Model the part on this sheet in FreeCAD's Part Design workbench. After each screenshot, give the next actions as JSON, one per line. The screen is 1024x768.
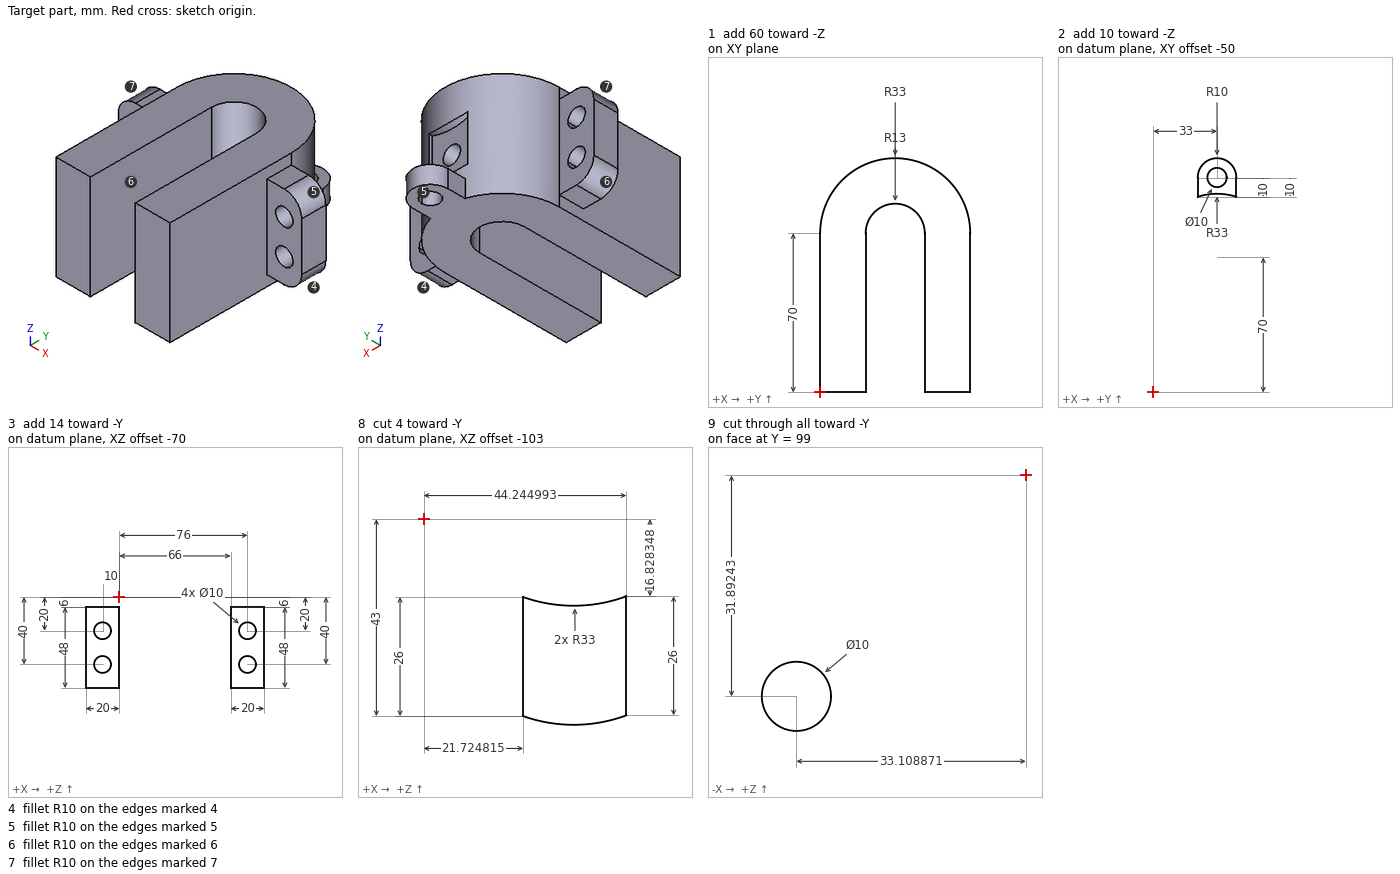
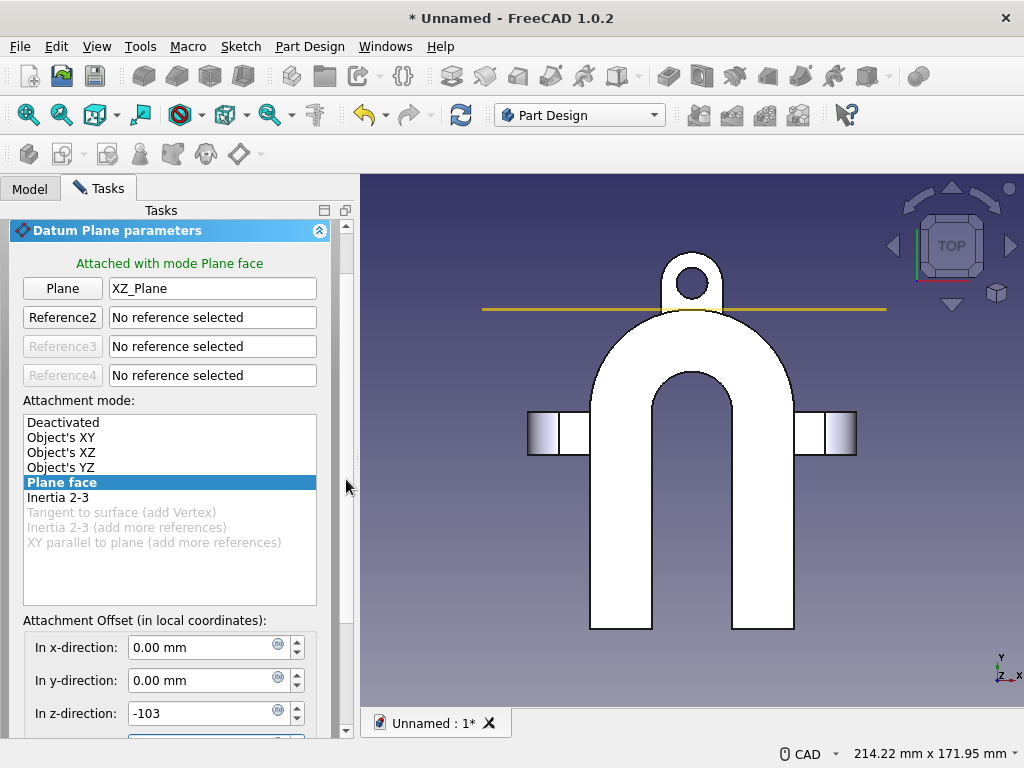
{"action": "left_click", "coordinate": [127, 249]}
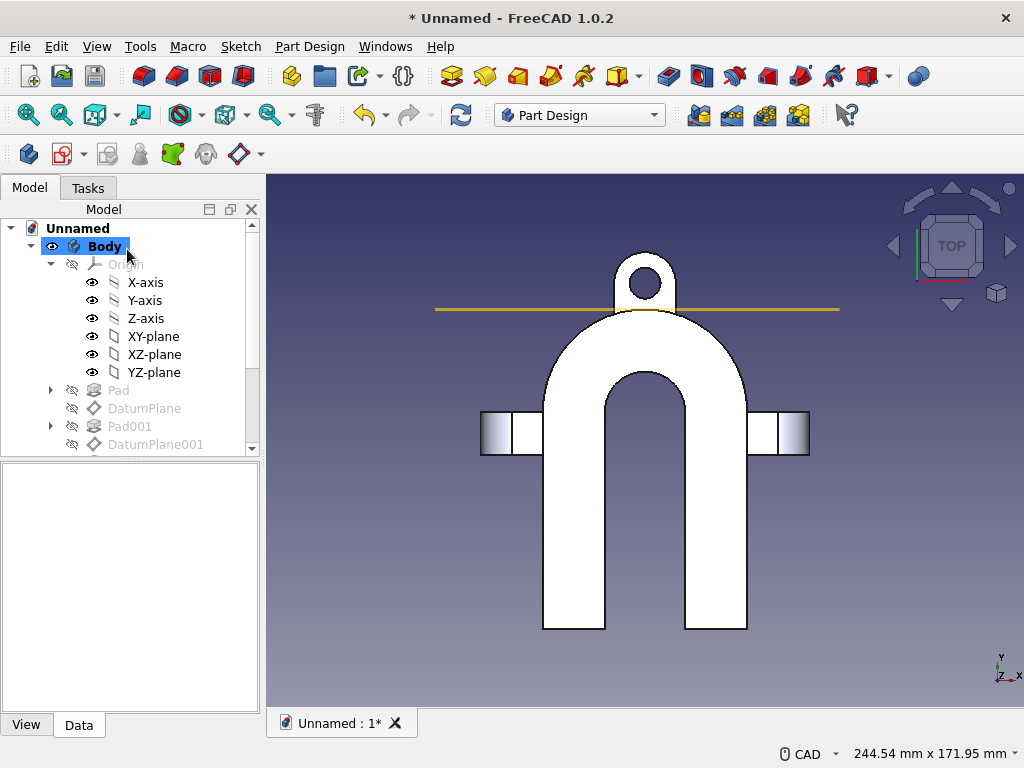
{"action": "scroll", "coordinate": [101, 332], "scroll_direction": "down", "scroll_amount": 3}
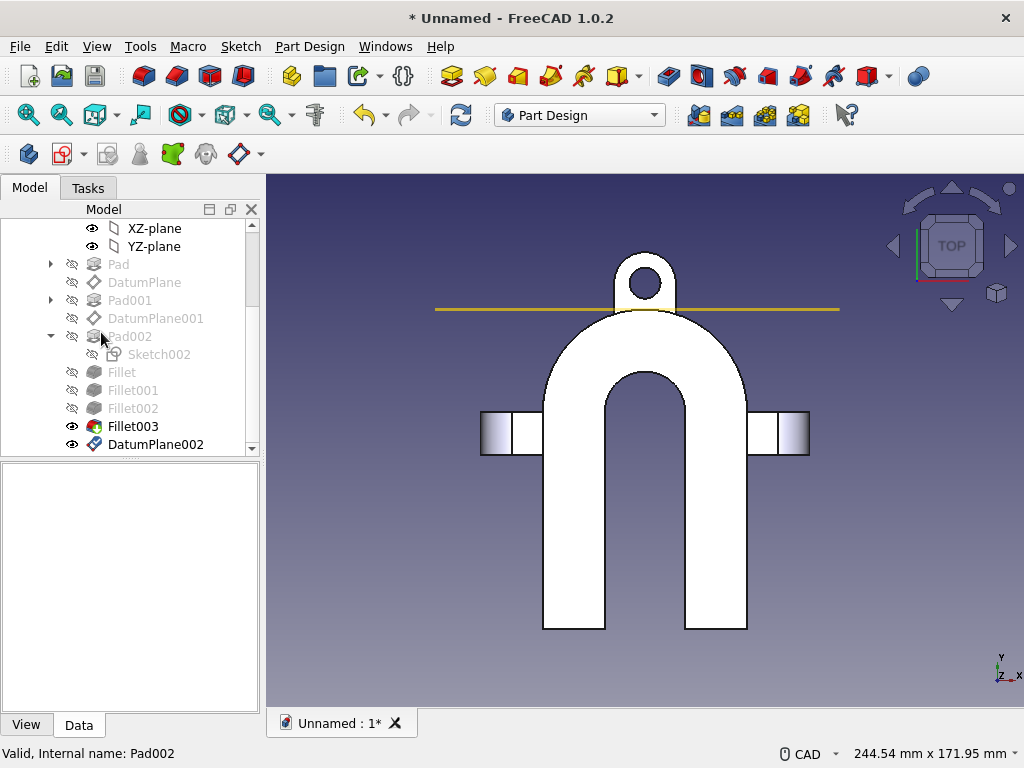
{"action": "left_click", "coordinate": [117, 444]}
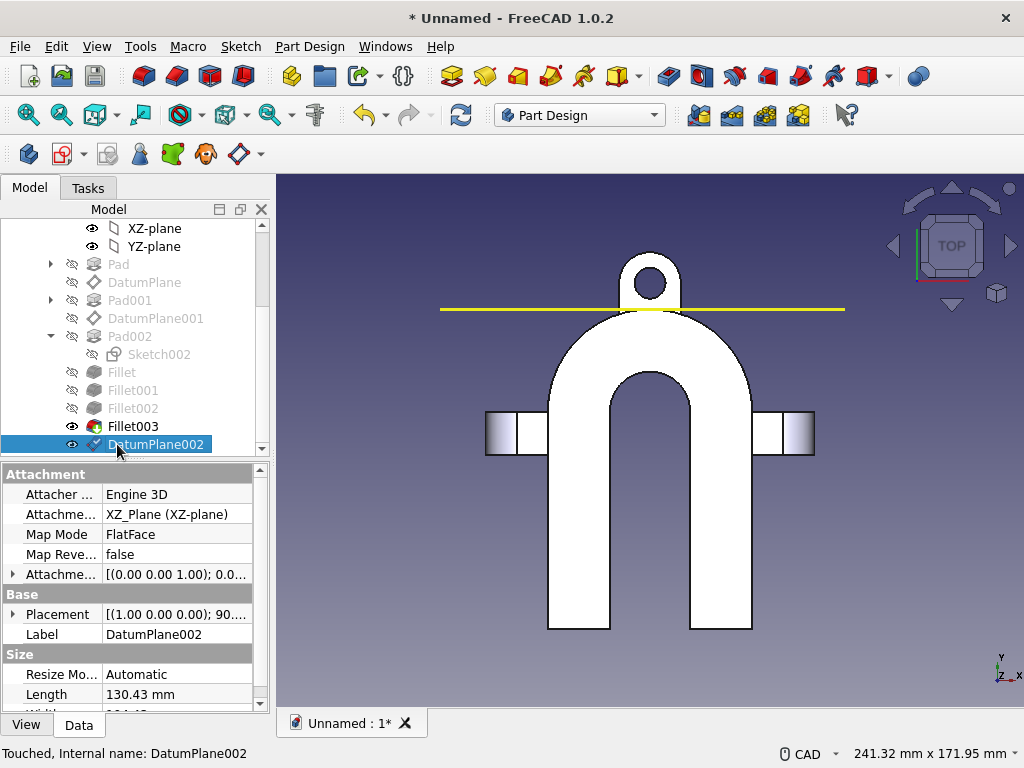
{"action": "left_click", "coordinate": [62, 154]}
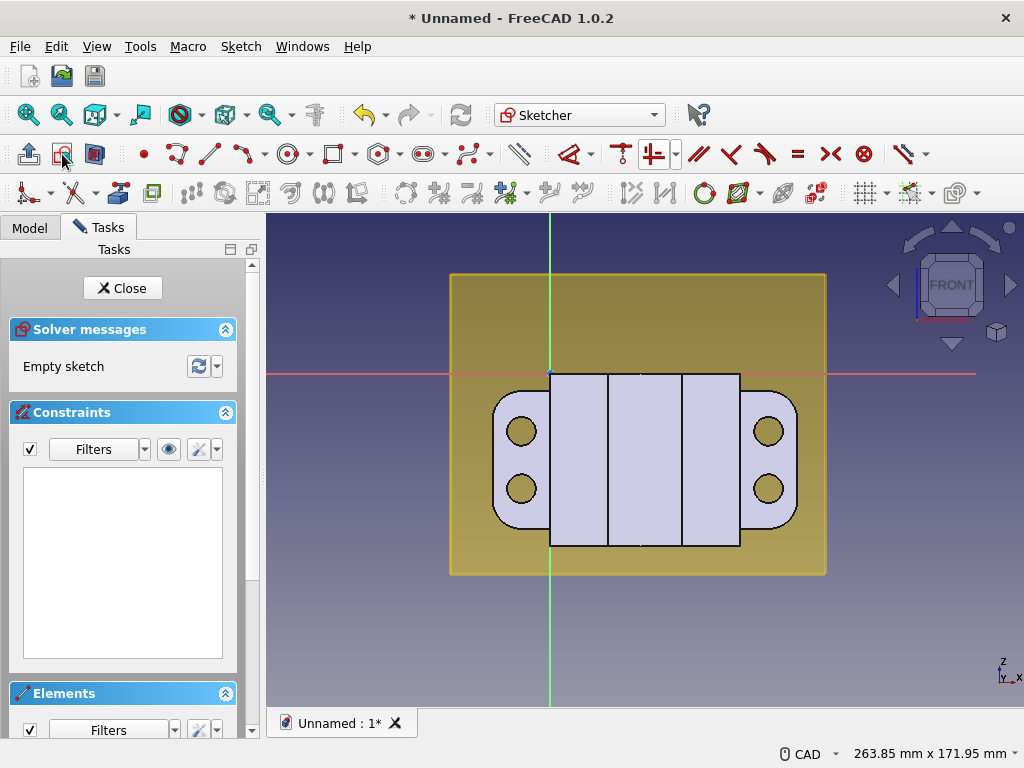
{"action": "left_click", "coordinate": [95, 154]}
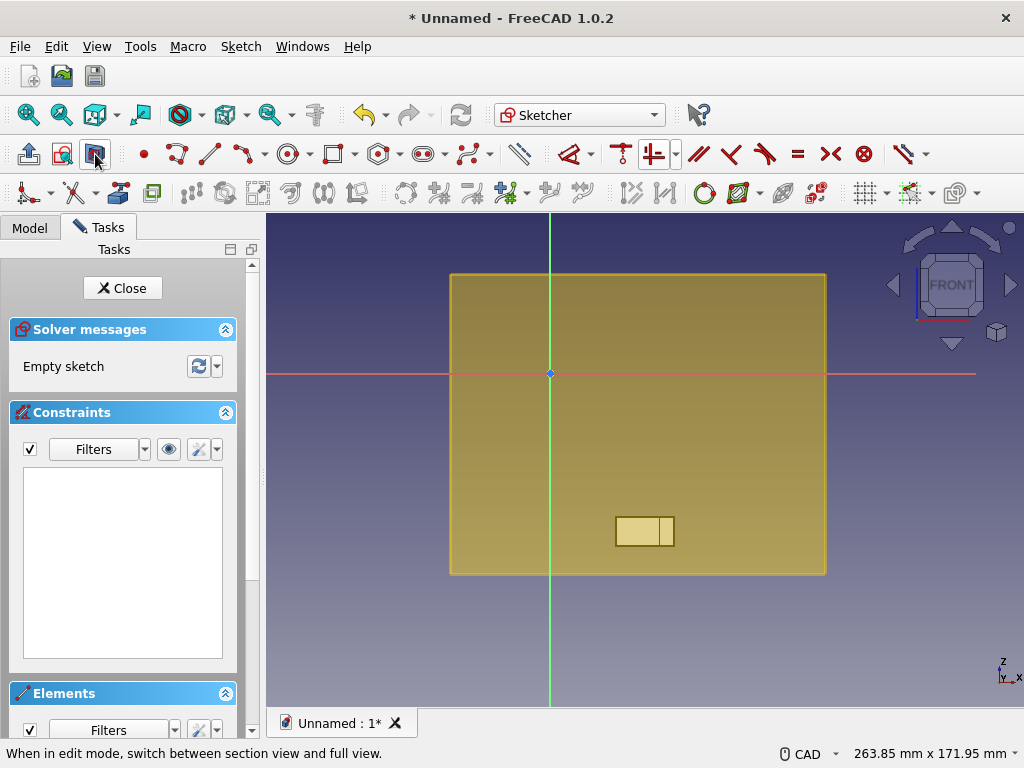
{"action": "scroll", "coordinate": [644, 421], "scroll_direction": "up", "scroll_amount": 4}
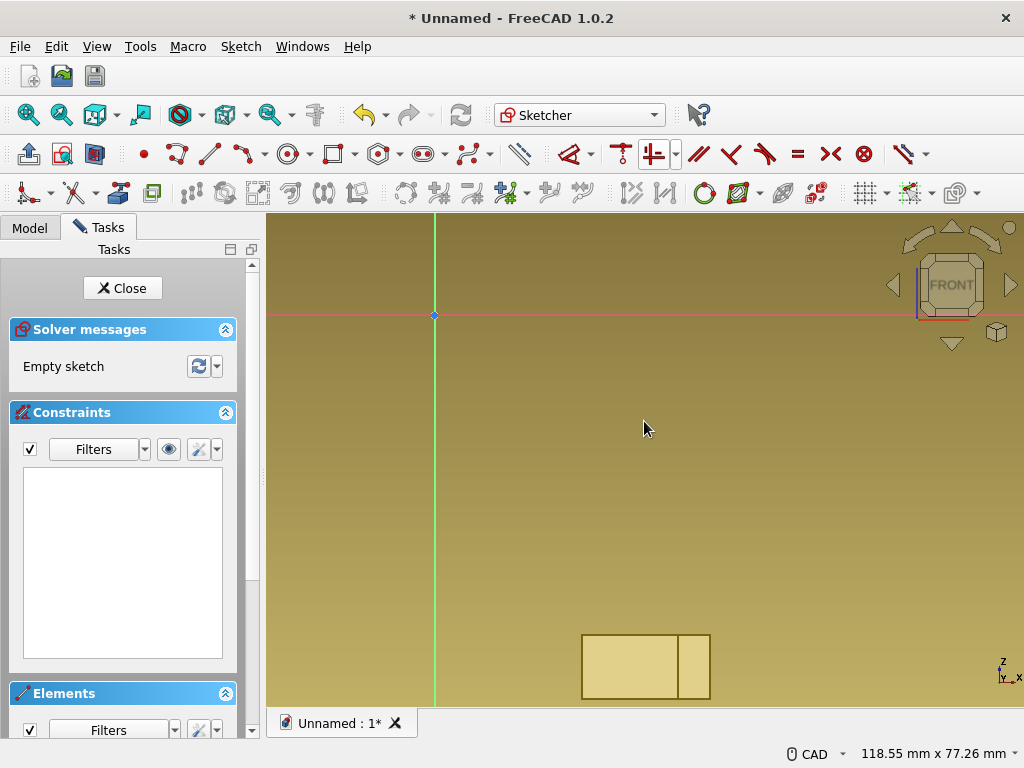
{"action": "key", "text": "g l"}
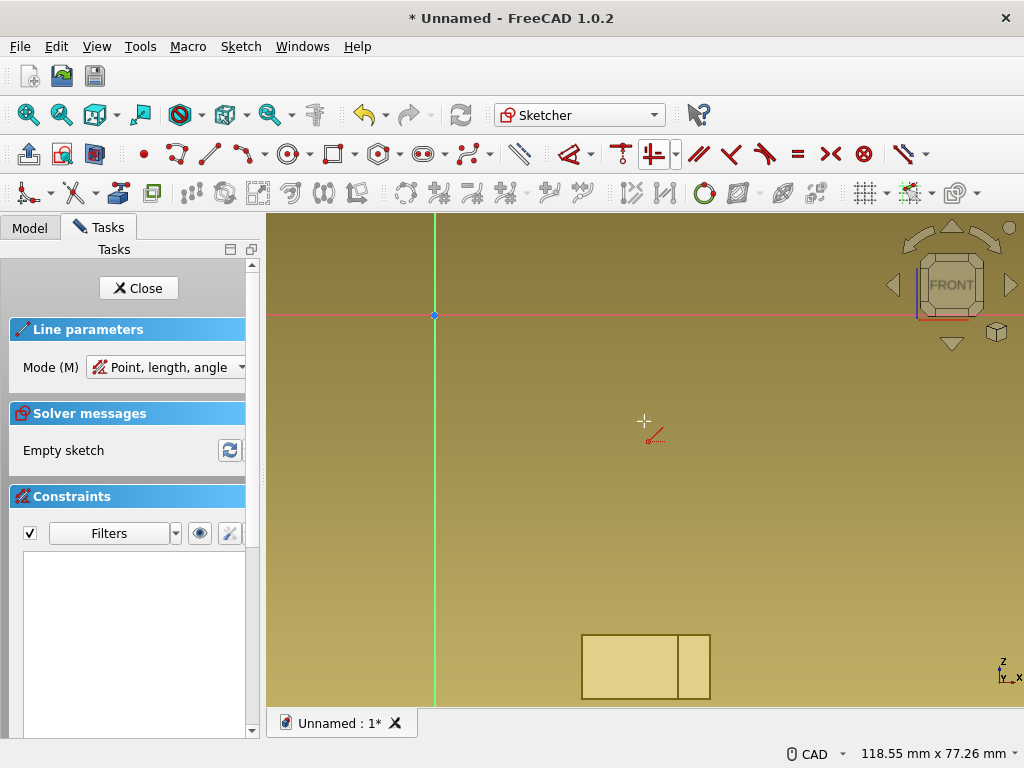
{"action": "left_click", "coordinate": [574, 590]}
{"action": "left_click", "coordinate": [574, 424]}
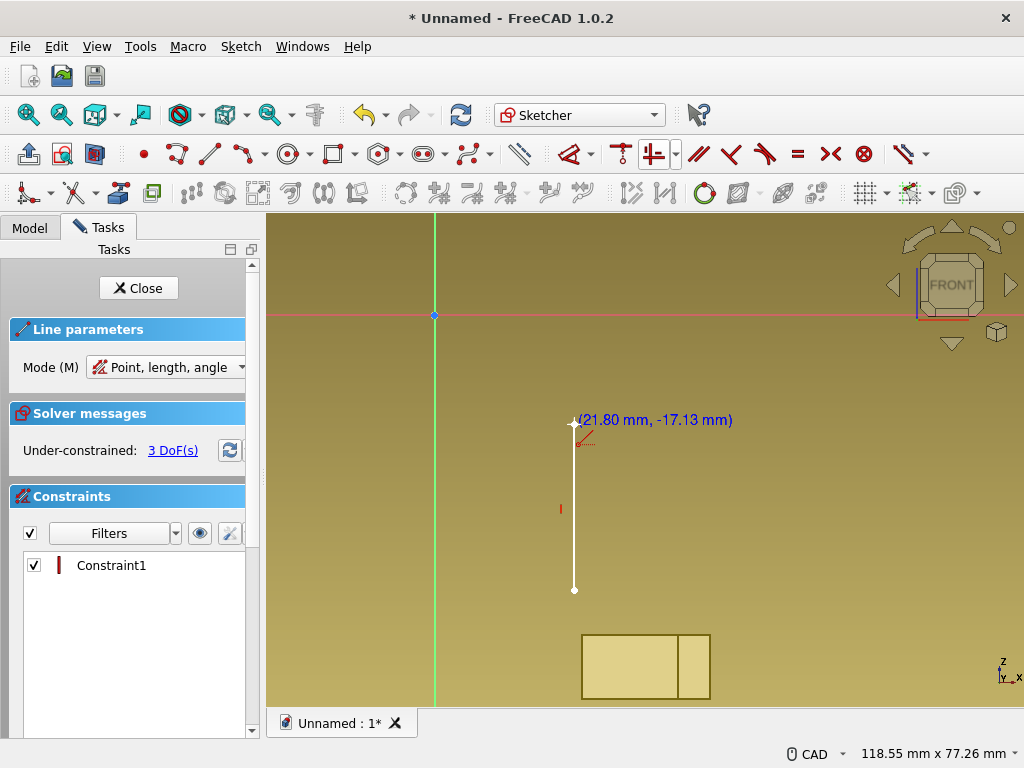
{"action": "left_click", "coordinate": [718, 423]}
{"action": "left_click", "coordinate": [718, 589]}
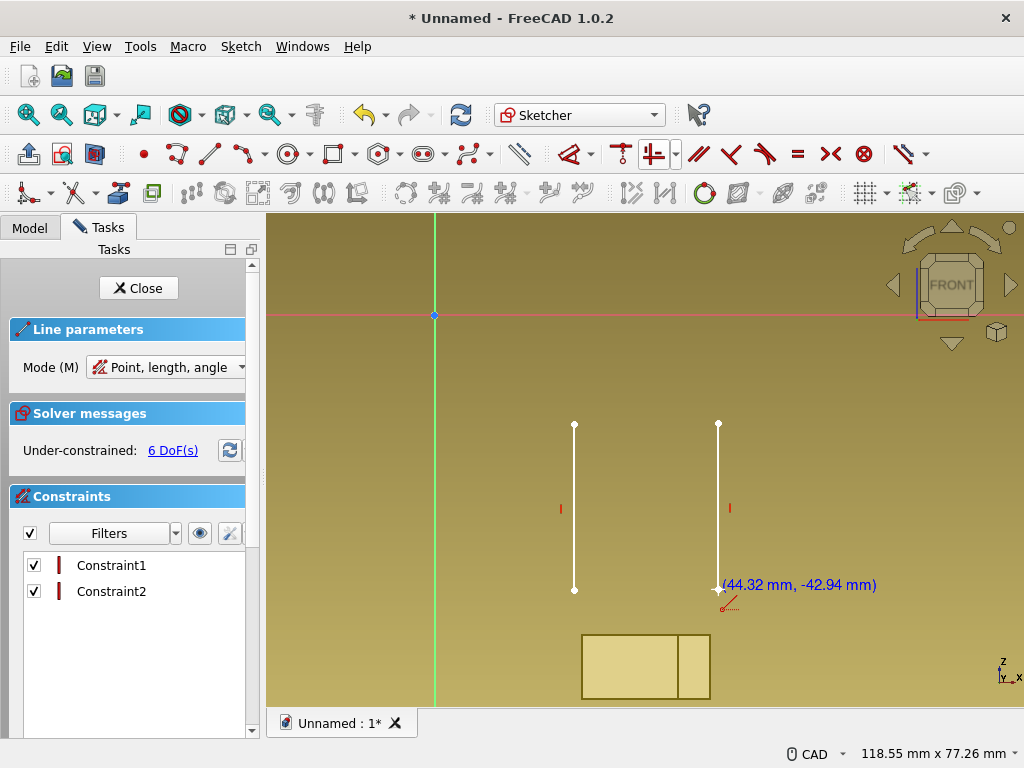
{"action": "left_click", "coordinate": [242, 154]}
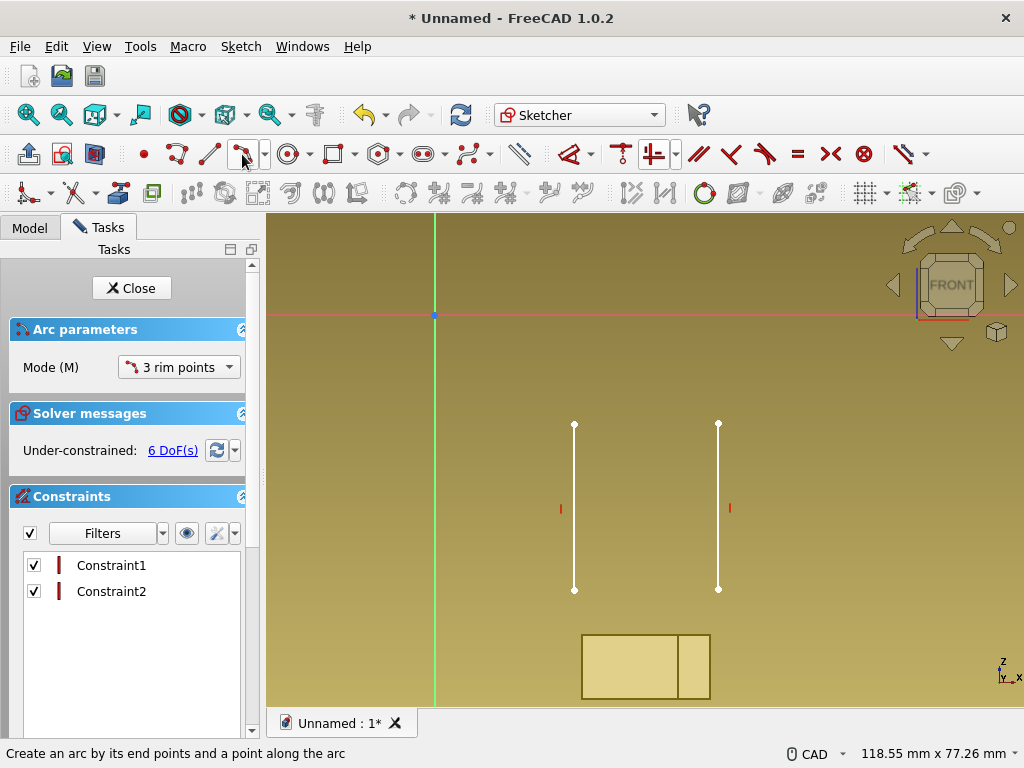
{"action": "left_click", "coordinate": [574, 425]}
{"action": "left_click", "coordinate": [718, 424]}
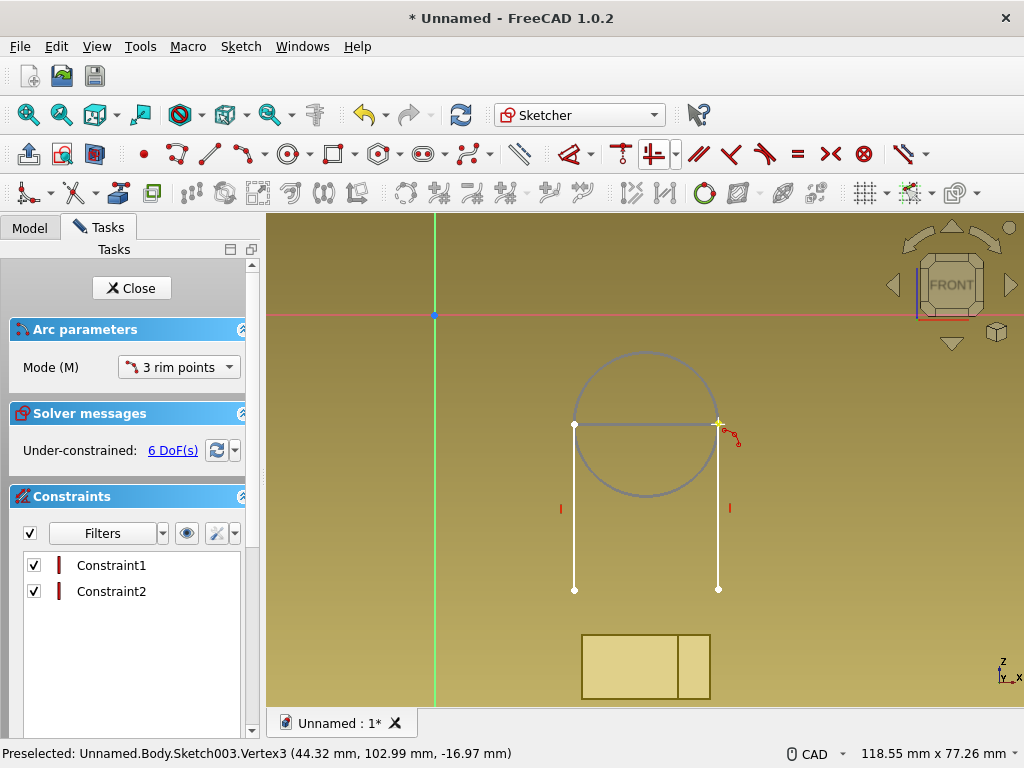
{"action": "scroll", "coordinate": [646, 436], "scroll_direction": "up", "scroll_amount": 2}